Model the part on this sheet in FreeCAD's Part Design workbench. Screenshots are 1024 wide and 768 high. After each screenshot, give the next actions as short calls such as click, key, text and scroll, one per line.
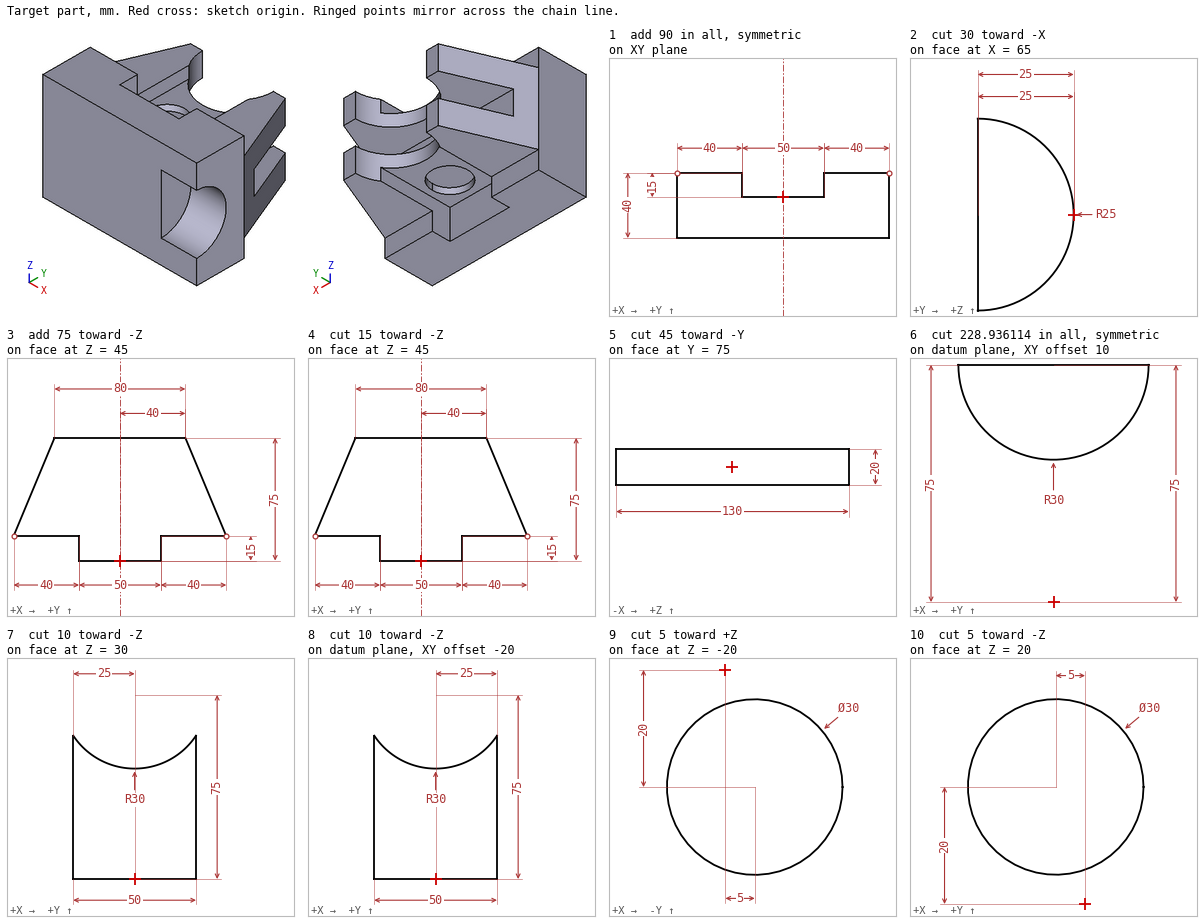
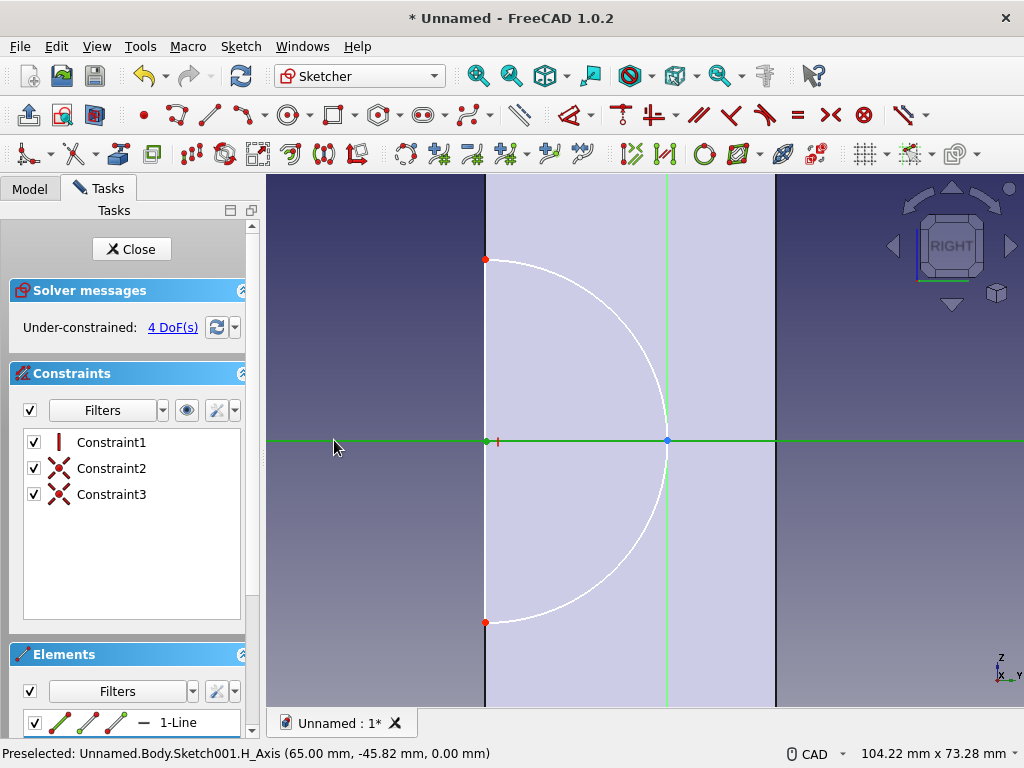
click(621, 116)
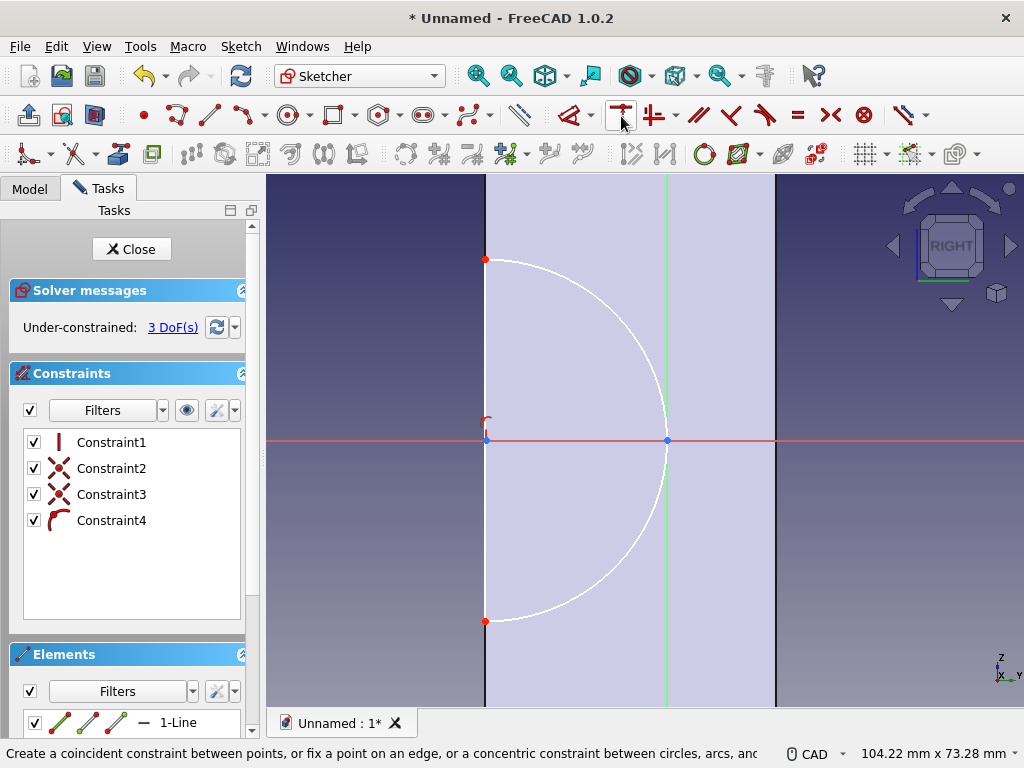
click(568, 116)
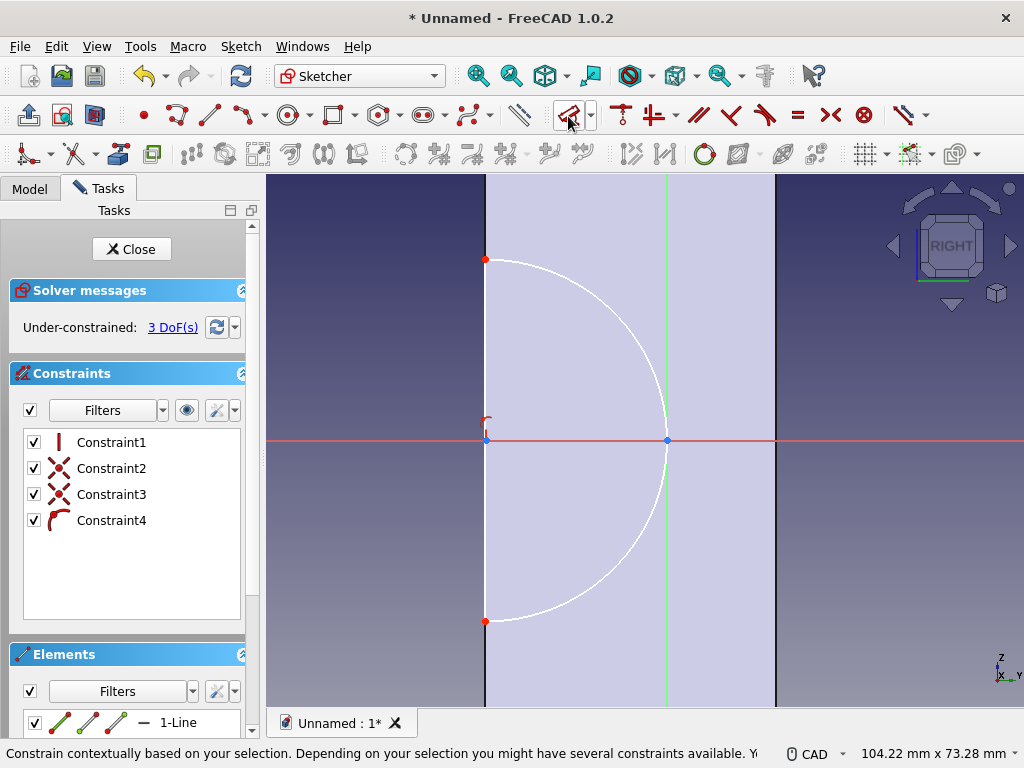
click(632, 547)
click(577, 633)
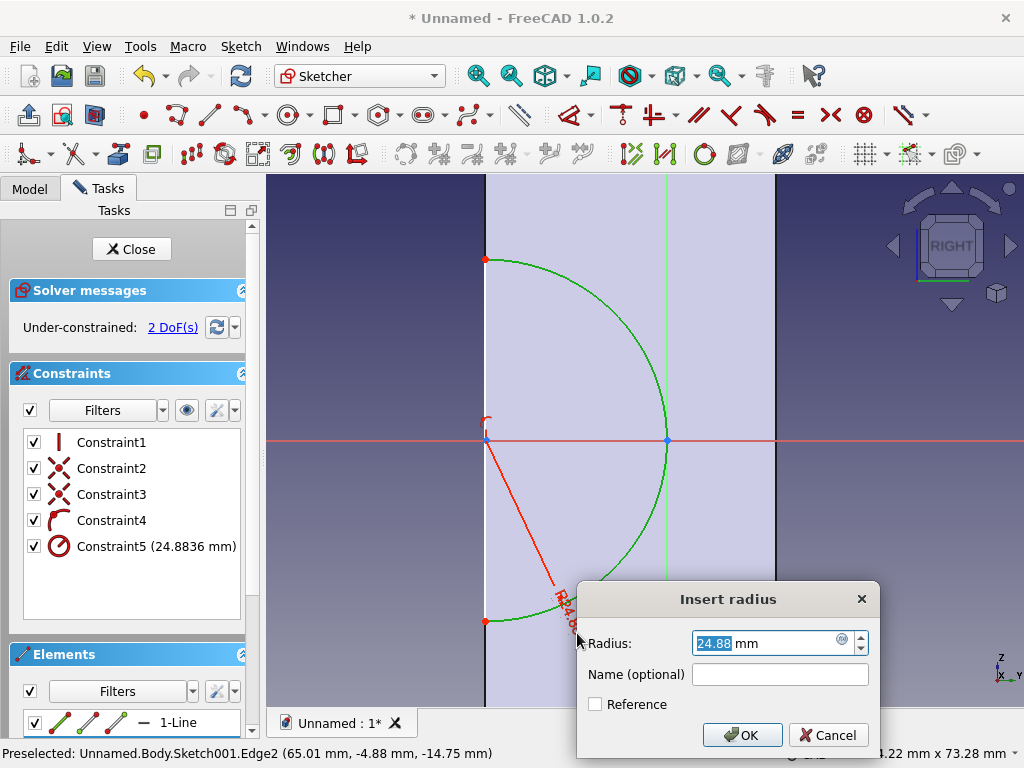
text(25)
key(Return)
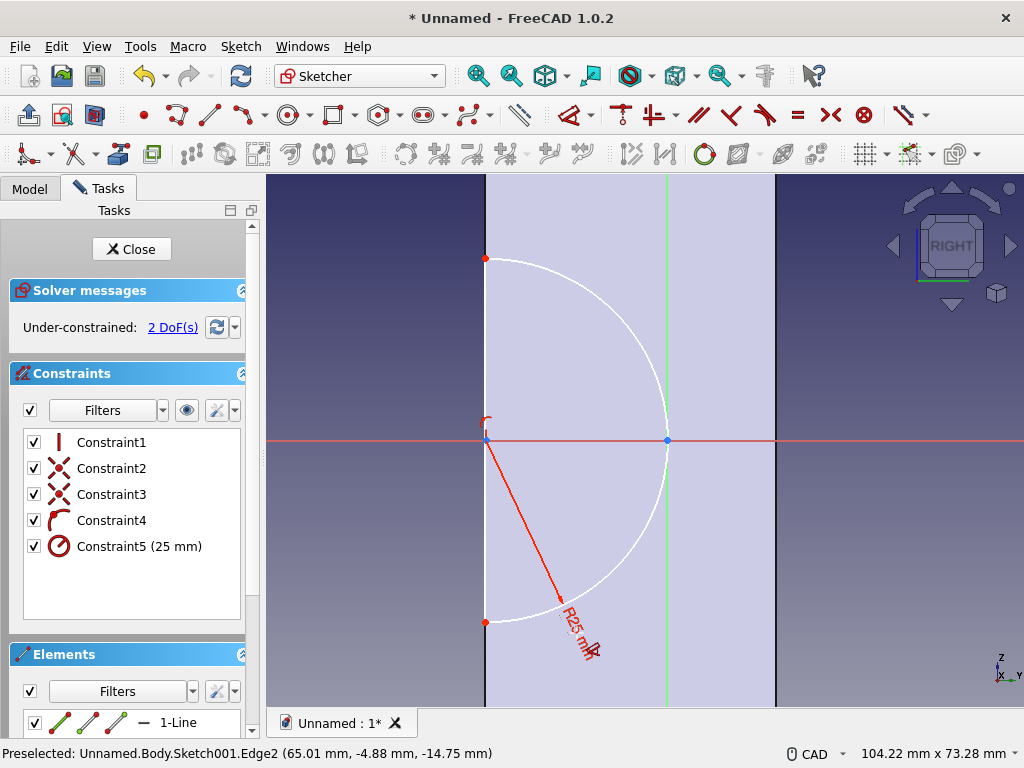
click(485, 259)
click(576, 225)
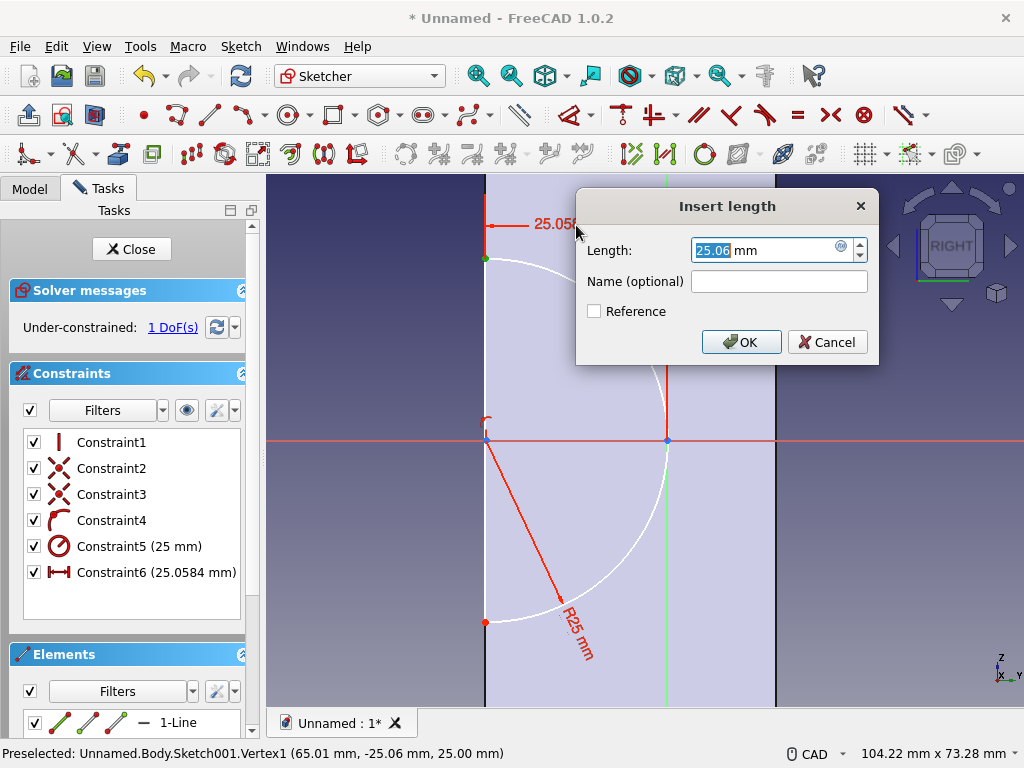
text(25)
key(Return)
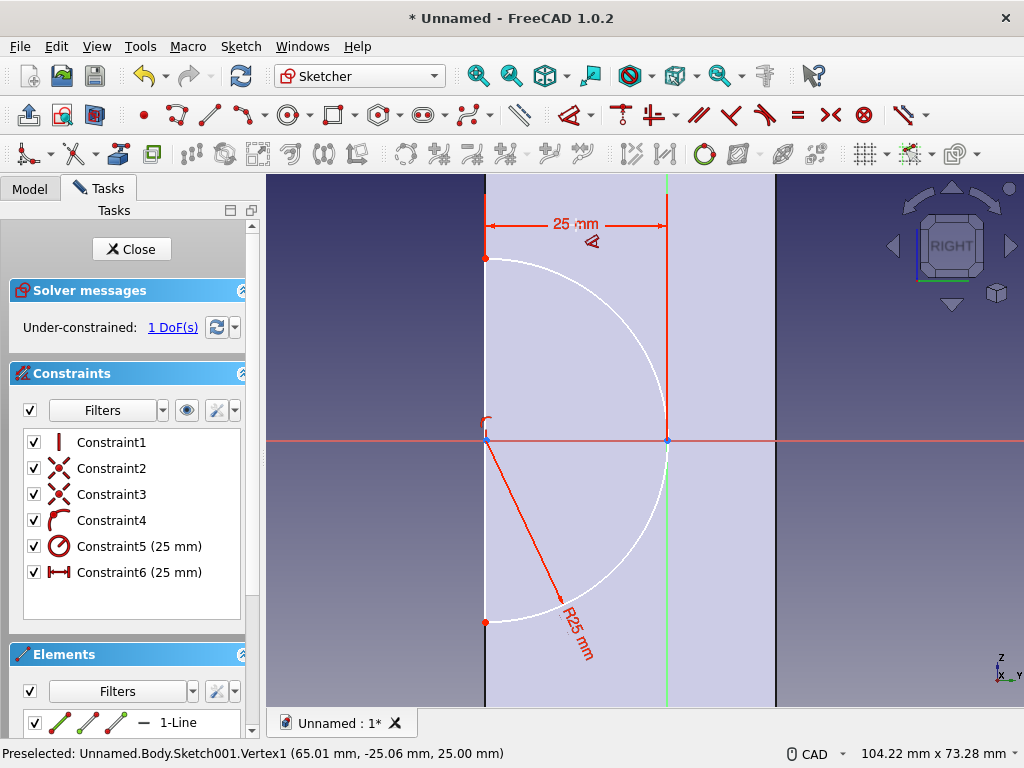
click(486, 440)
click(577, 474)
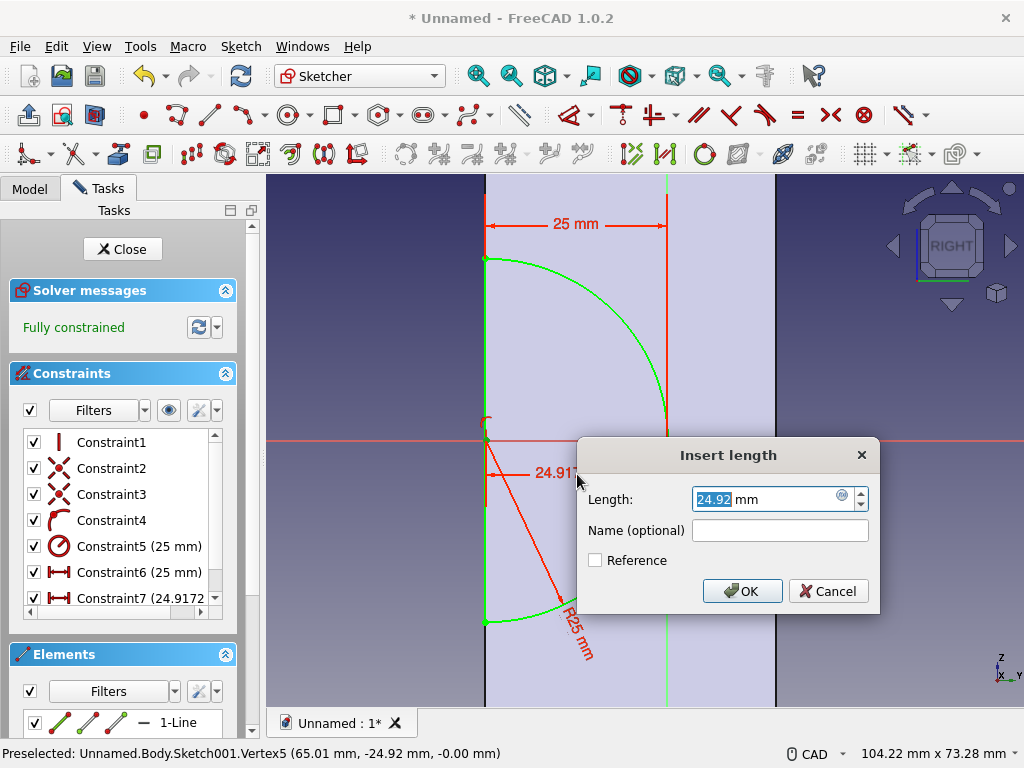
text(25)
key(Return)
key(Escape)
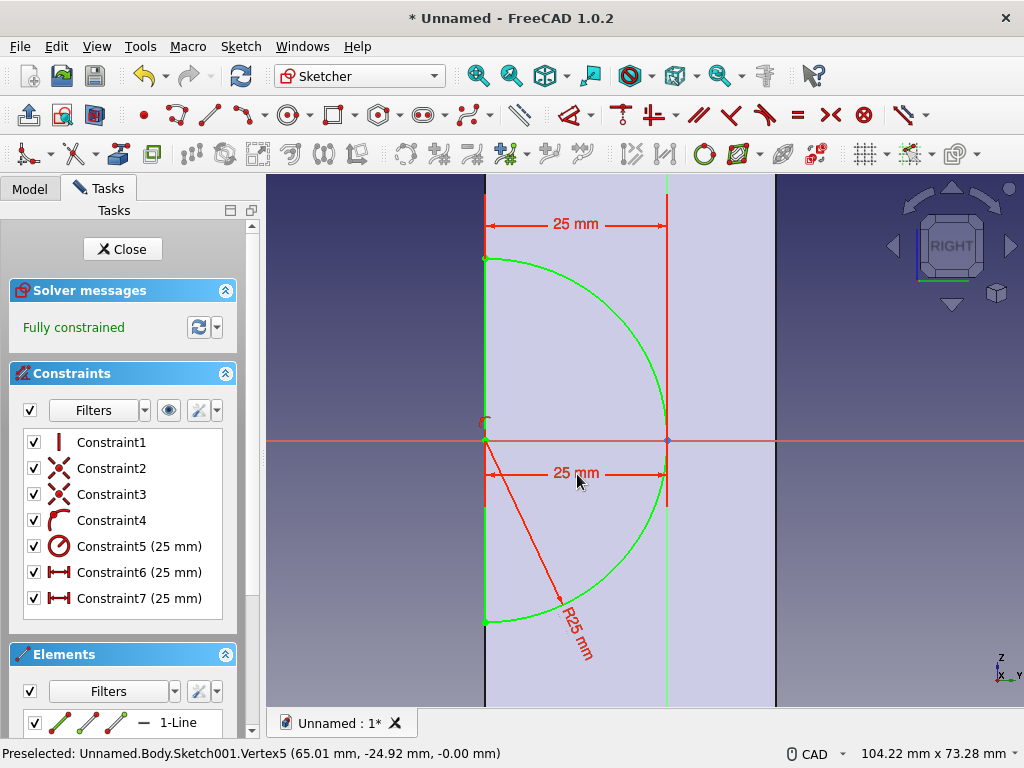
click(123, 249)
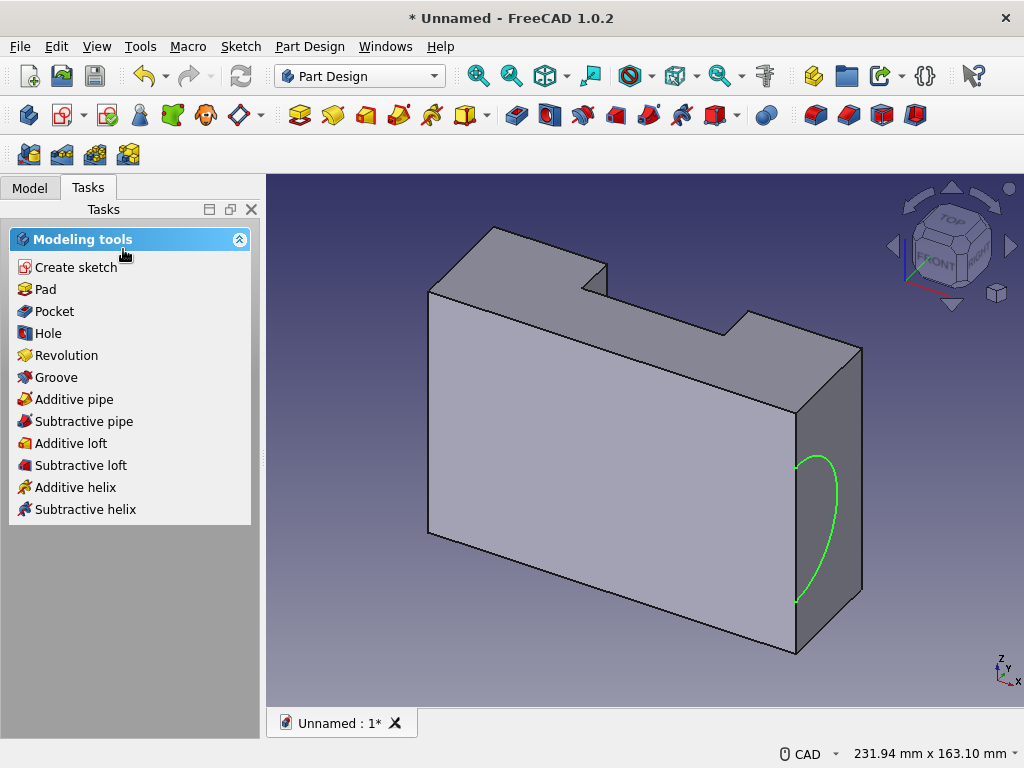
click(517, 116)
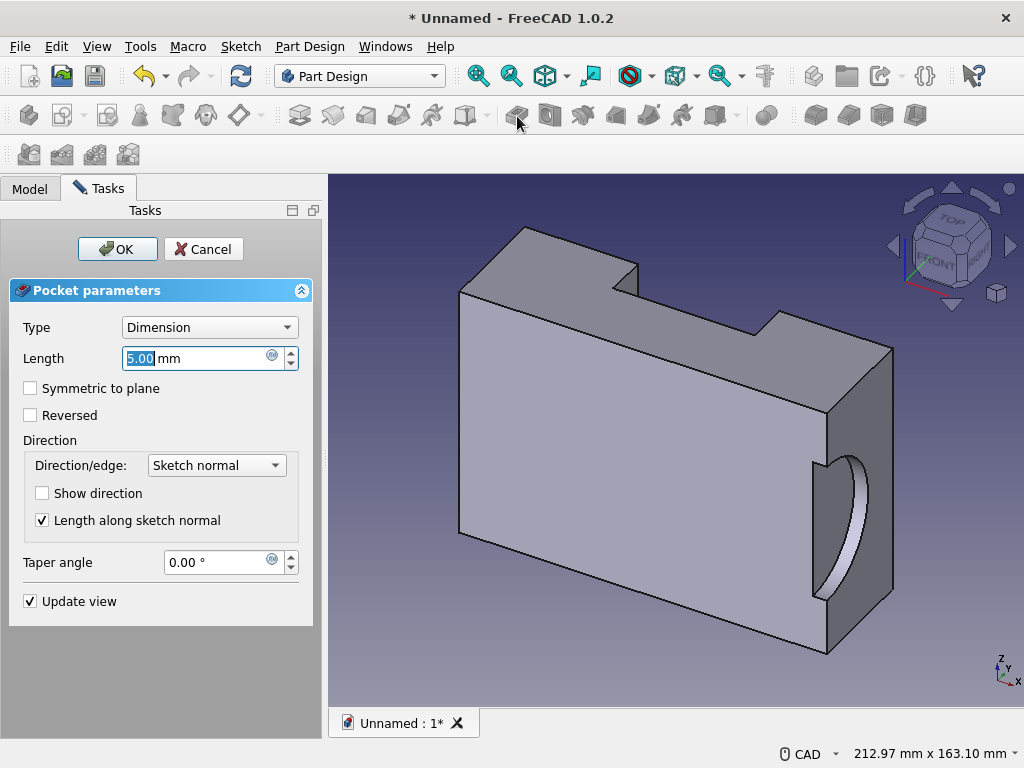
text(30)
key(Tab)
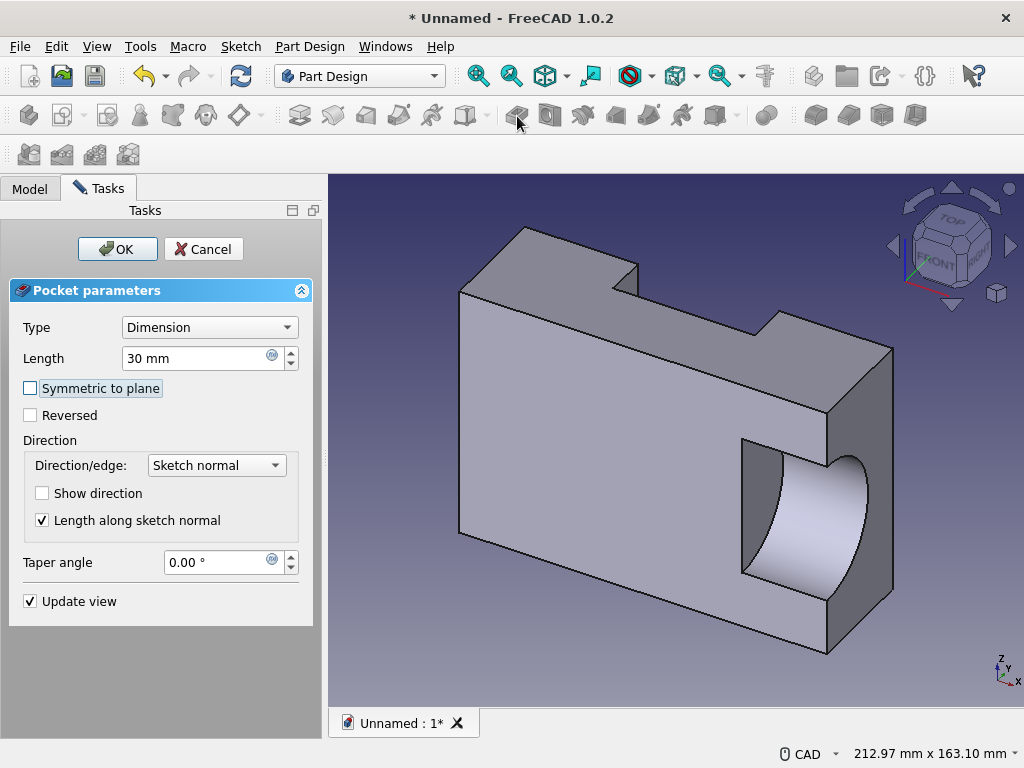
click(118, 249)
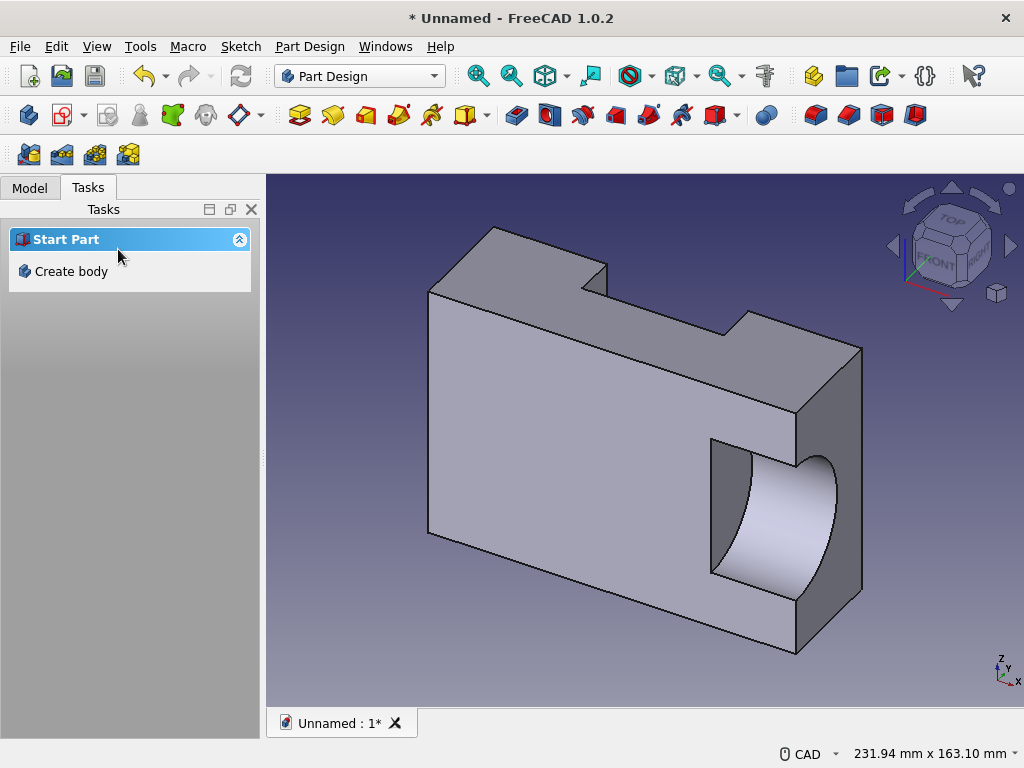
click(741, 363)